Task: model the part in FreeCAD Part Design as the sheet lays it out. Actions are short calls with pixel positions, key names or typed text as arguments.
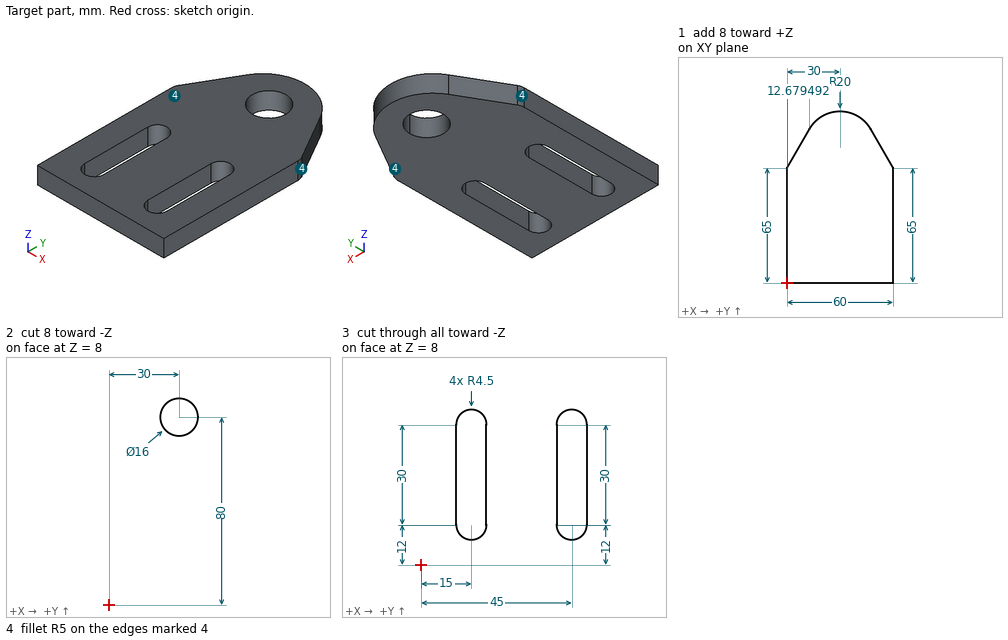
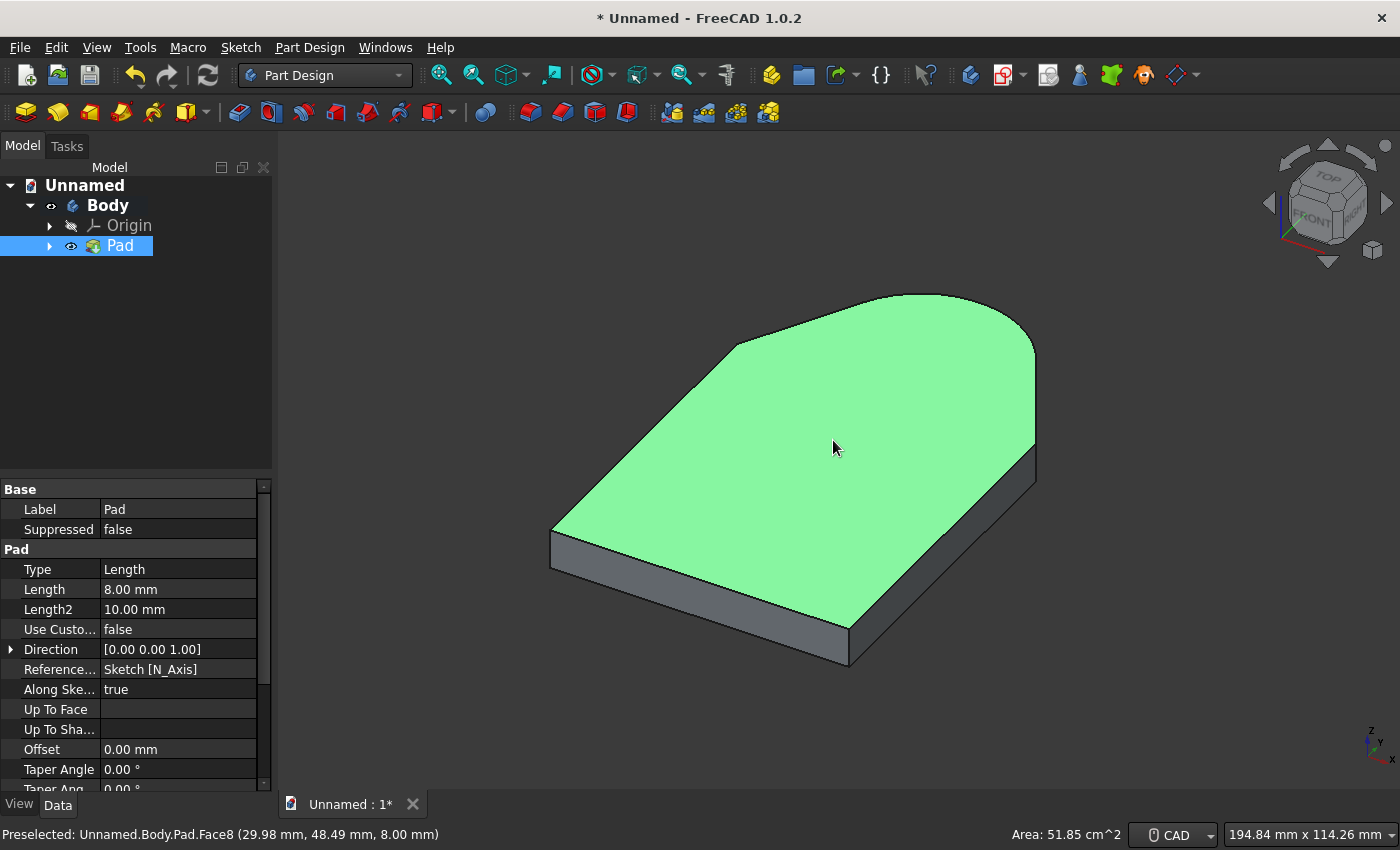
click(1004, 76)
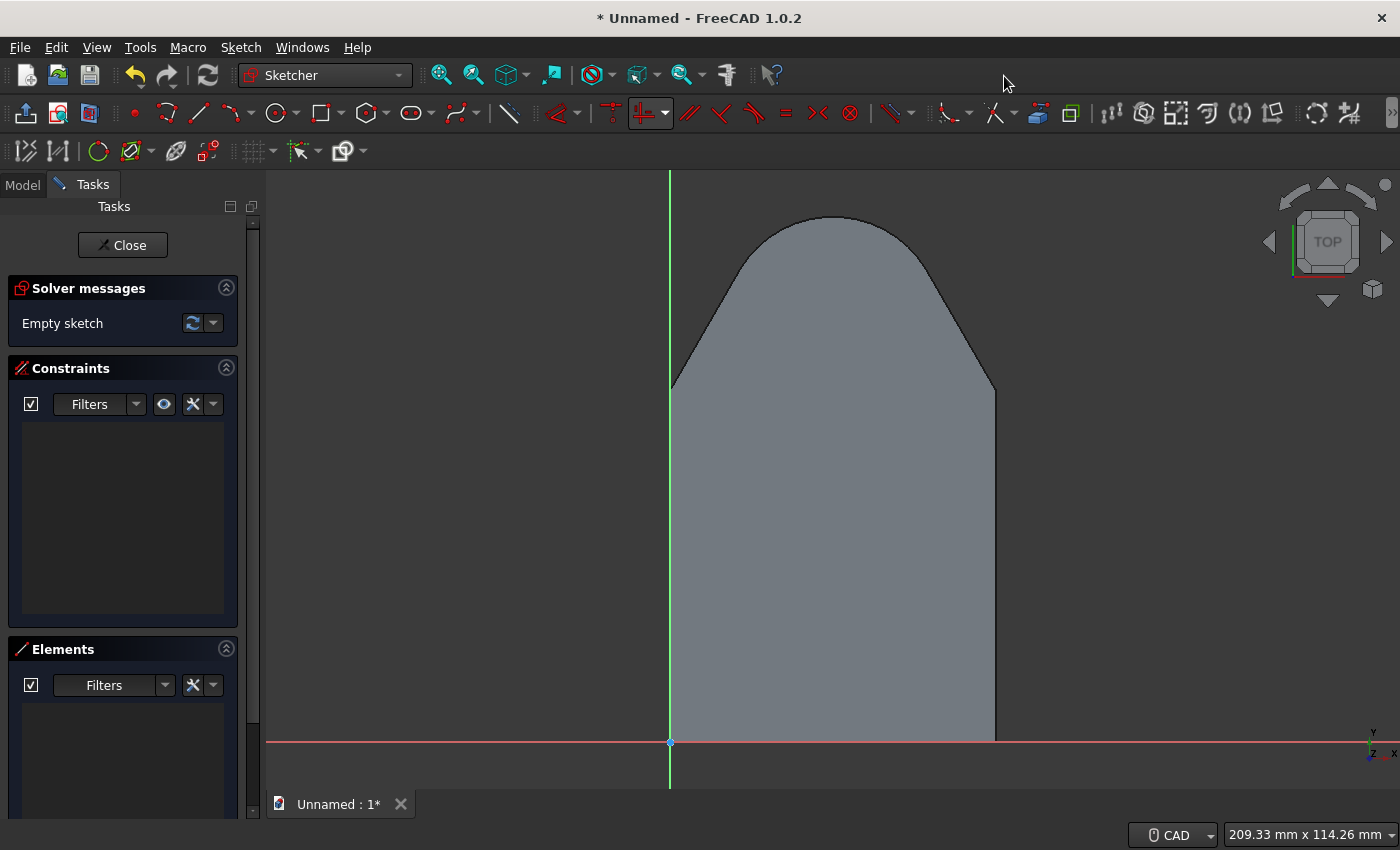
scroll(850, 265, up, 8)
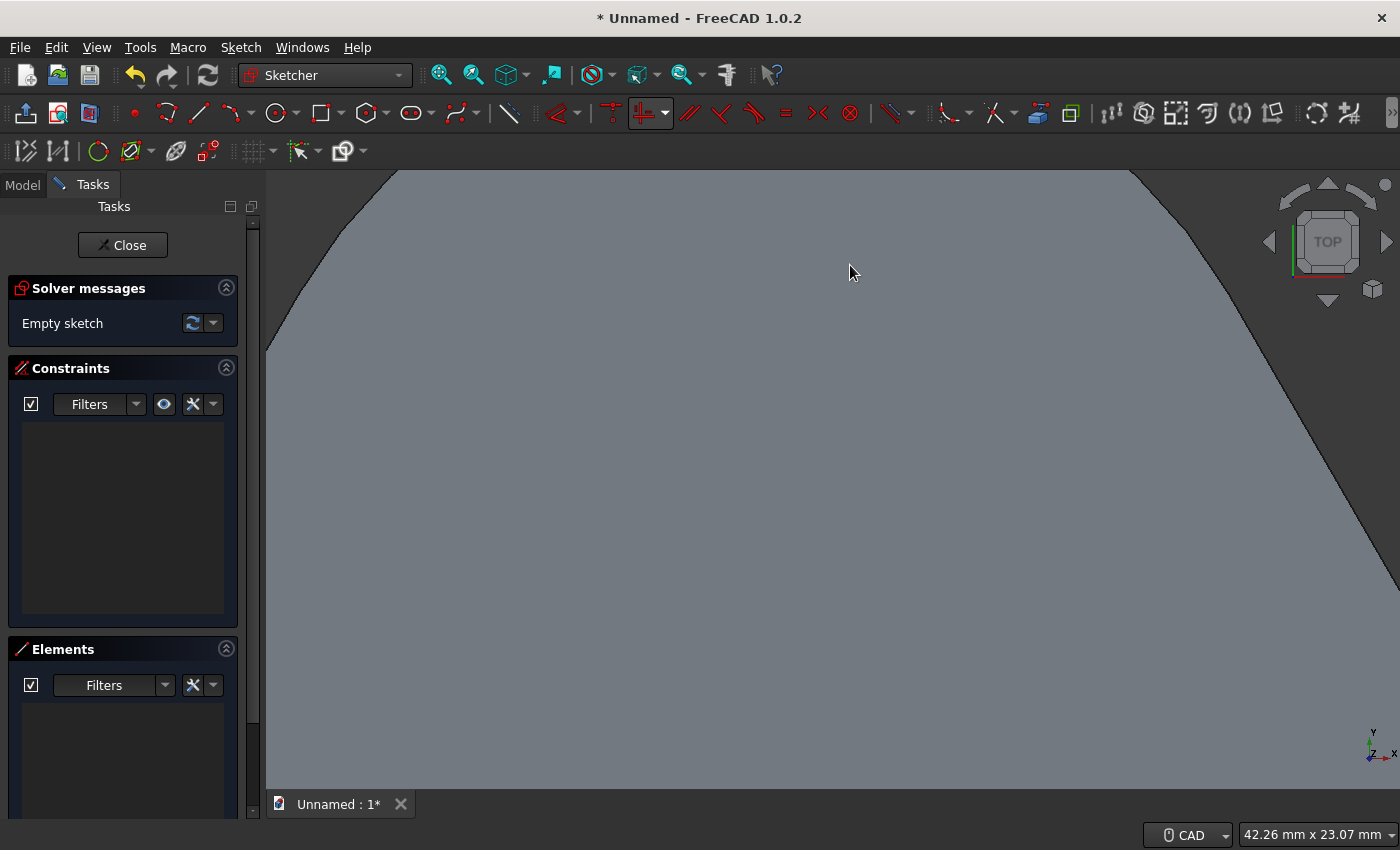
click(276, 114)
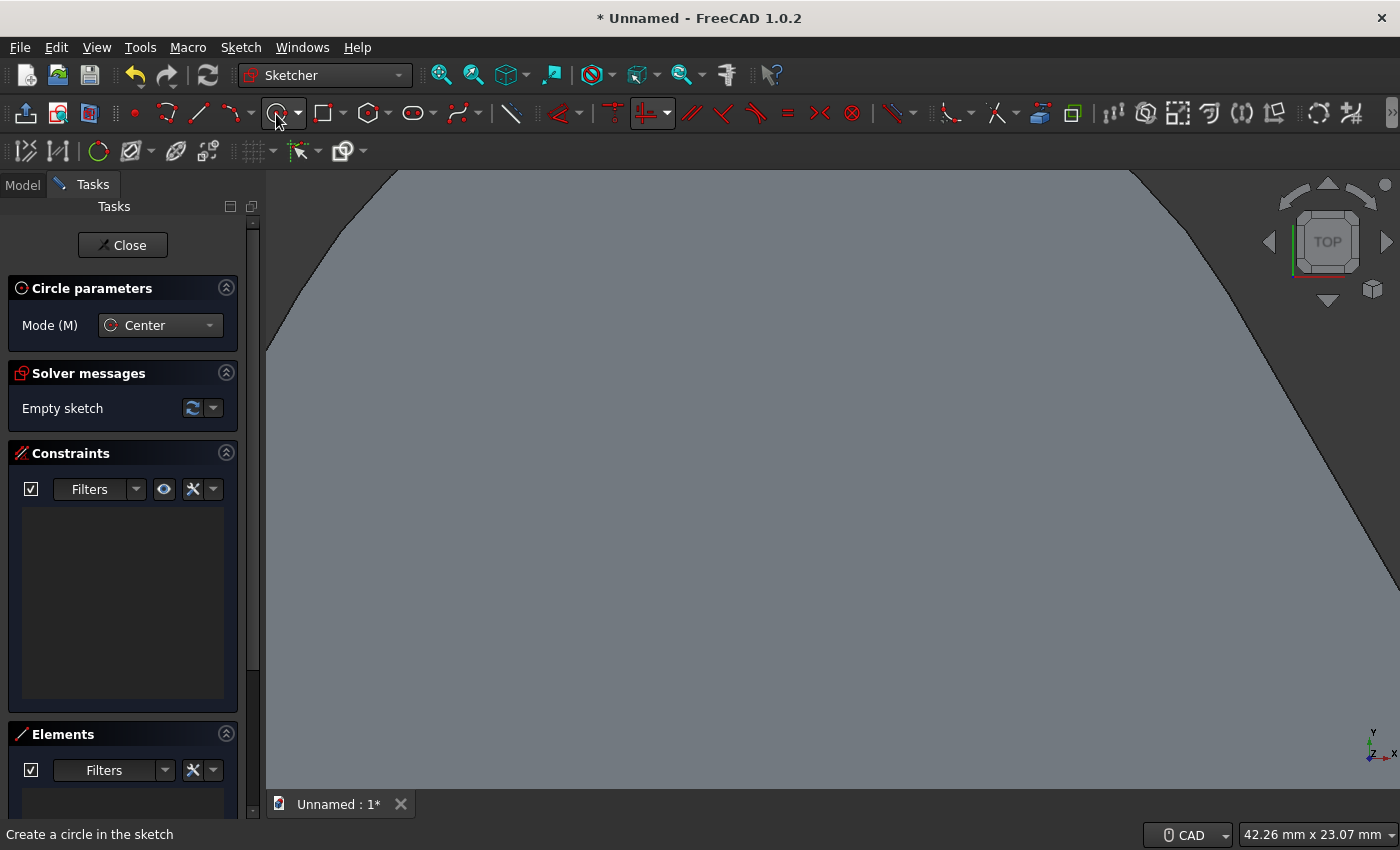
click(764, 480)
move(916, 329)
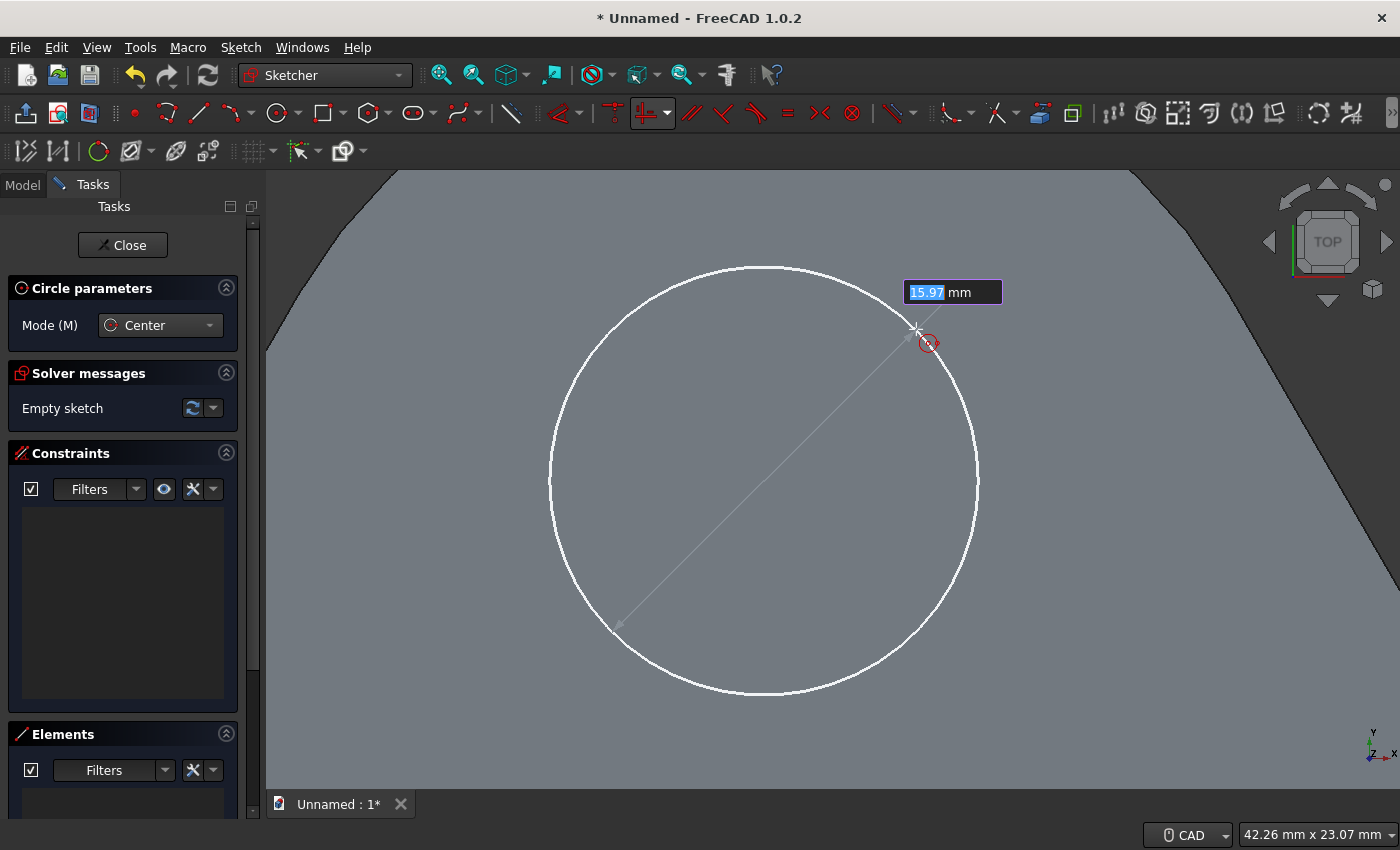
text(16)
key(Return)
key(Escape)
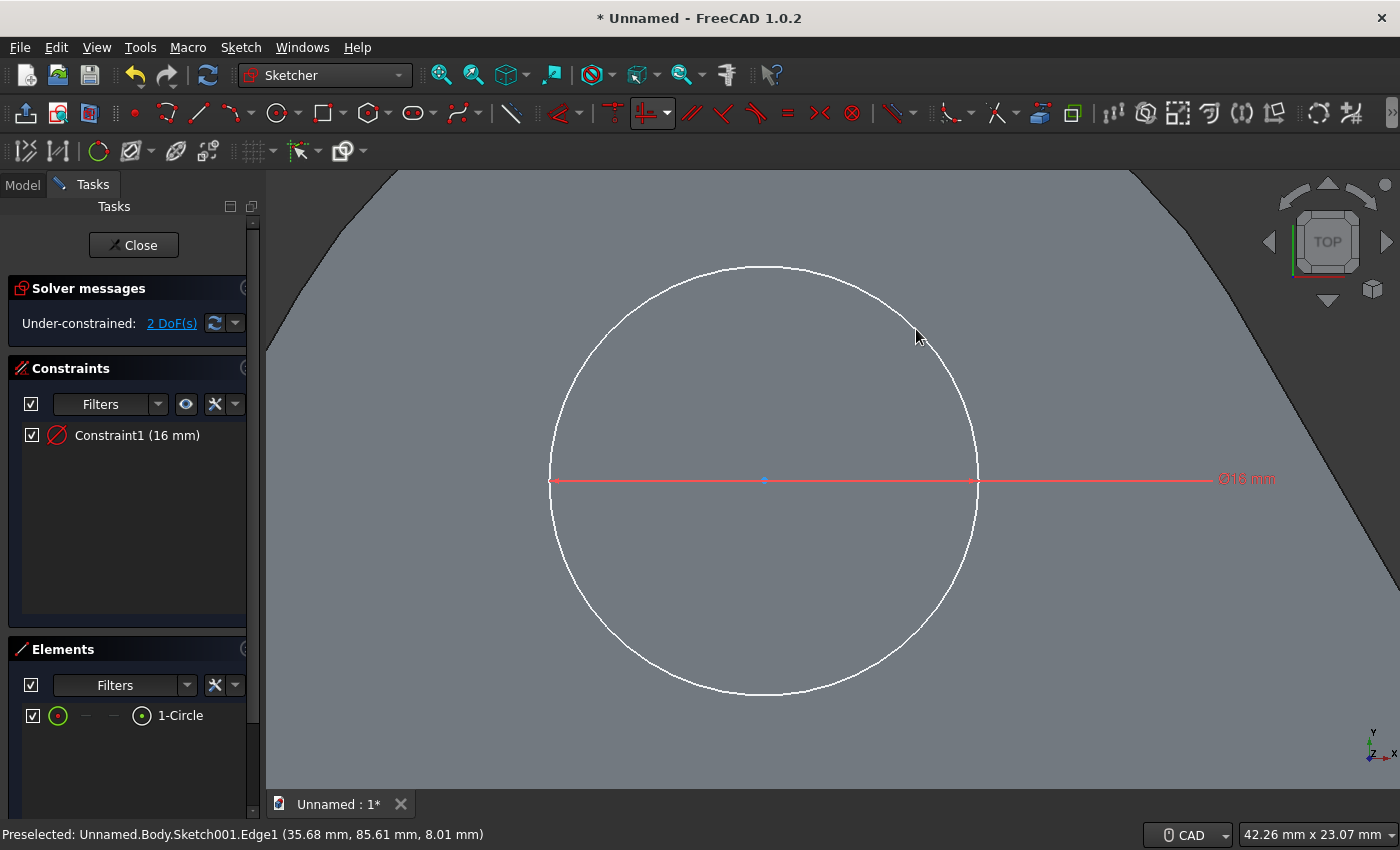
click(558, 114)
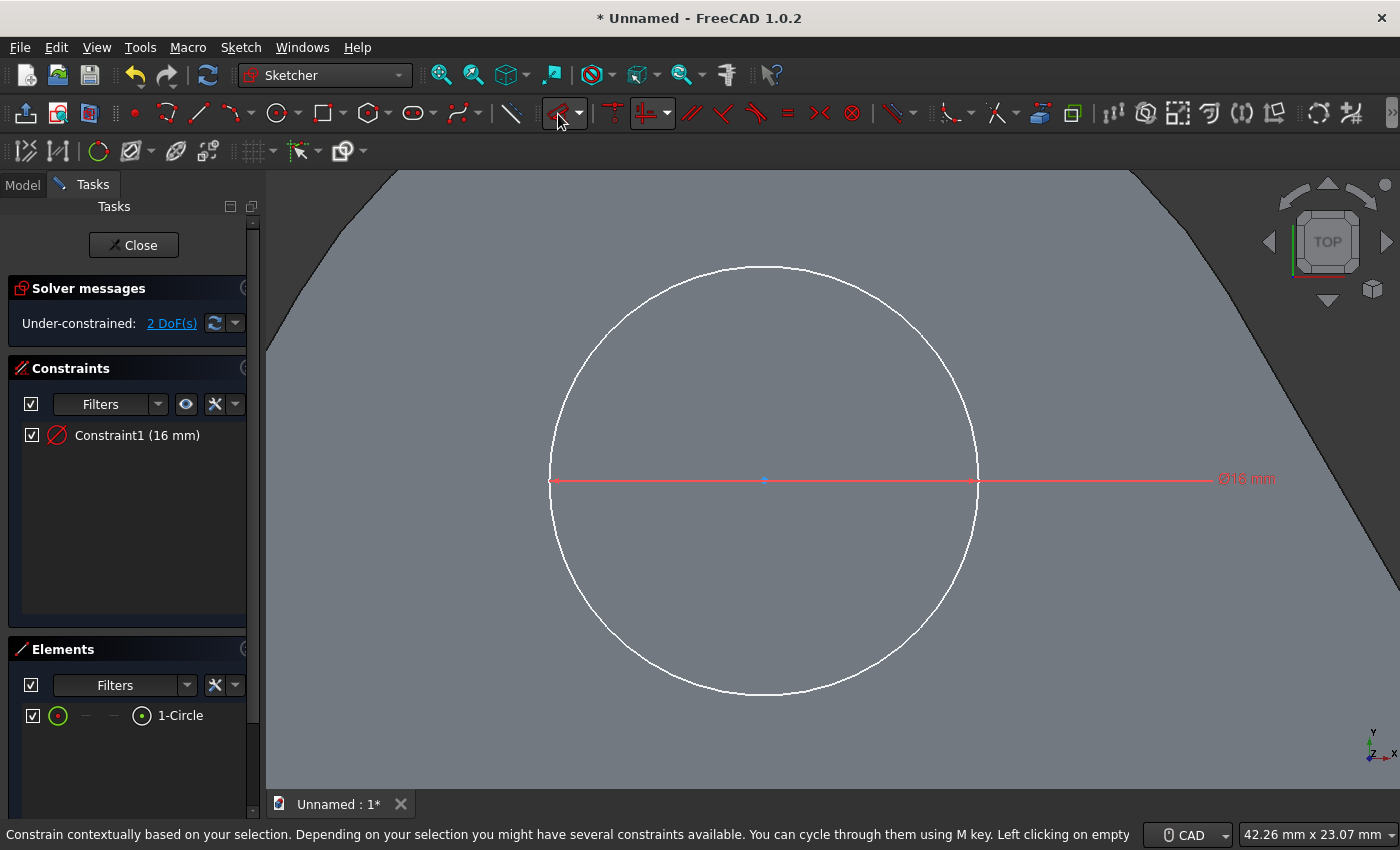
click(764, 481)
click(529, 447)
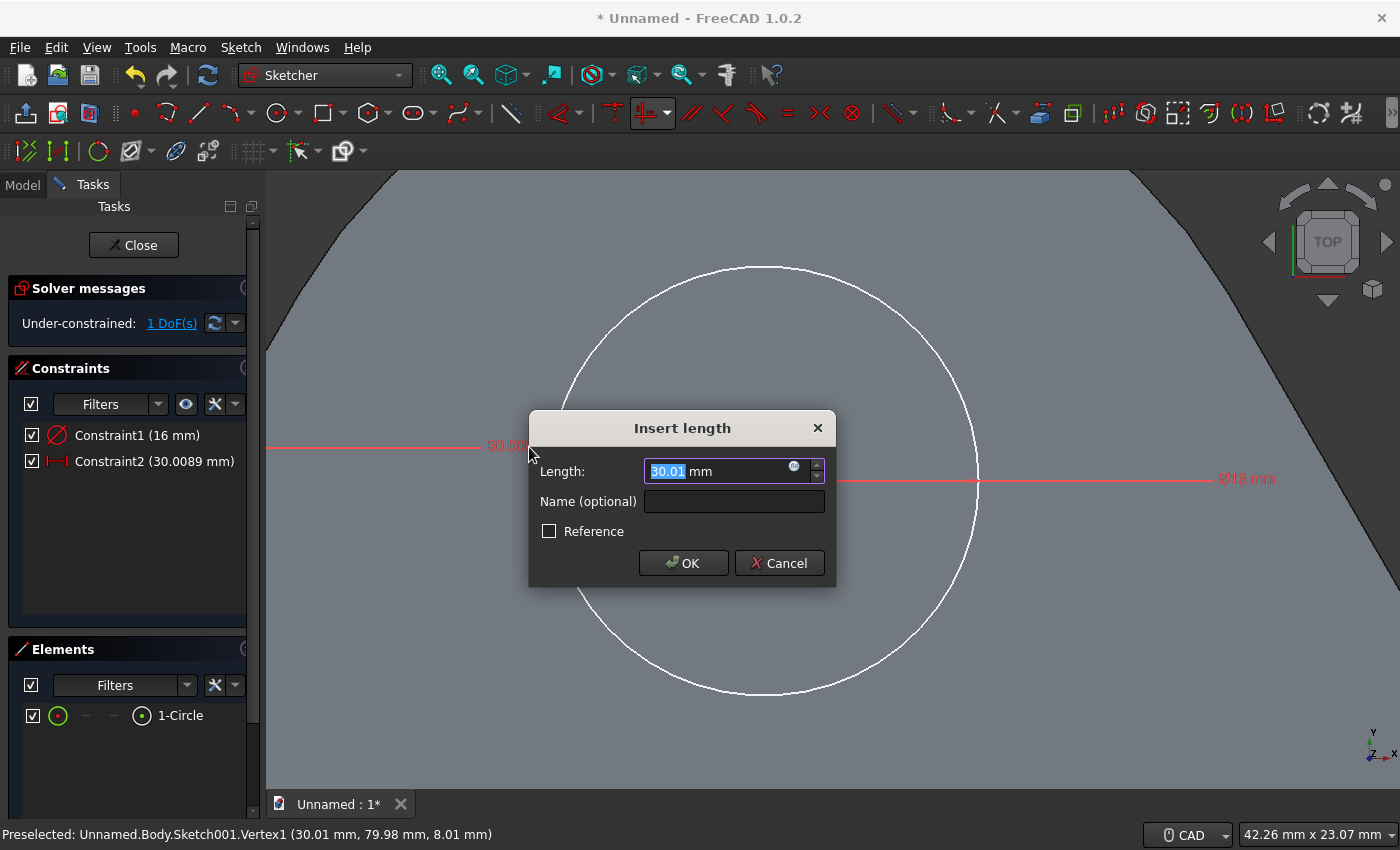
text(30)
key(Return)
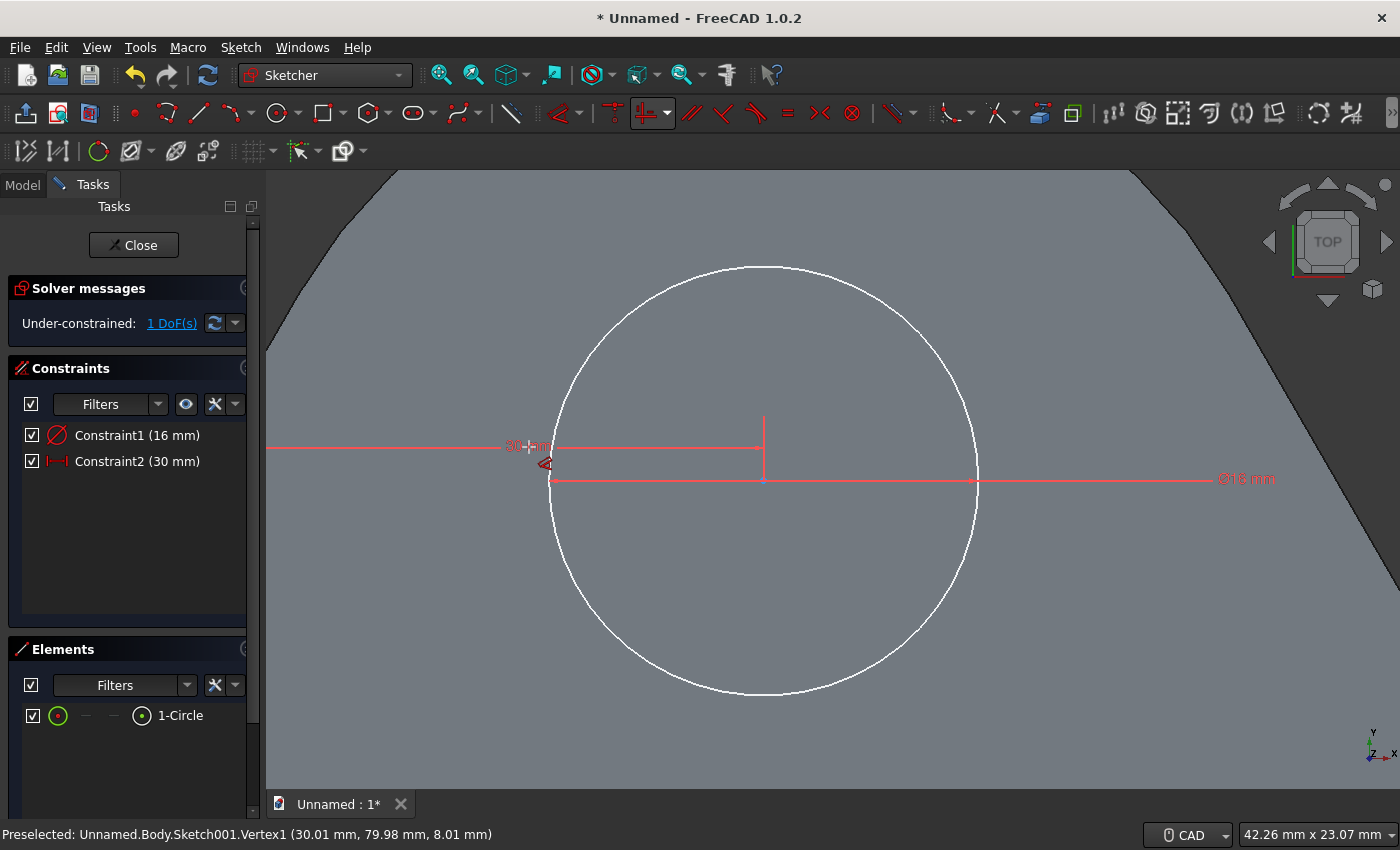
click(764, 481)
click(798, 621)